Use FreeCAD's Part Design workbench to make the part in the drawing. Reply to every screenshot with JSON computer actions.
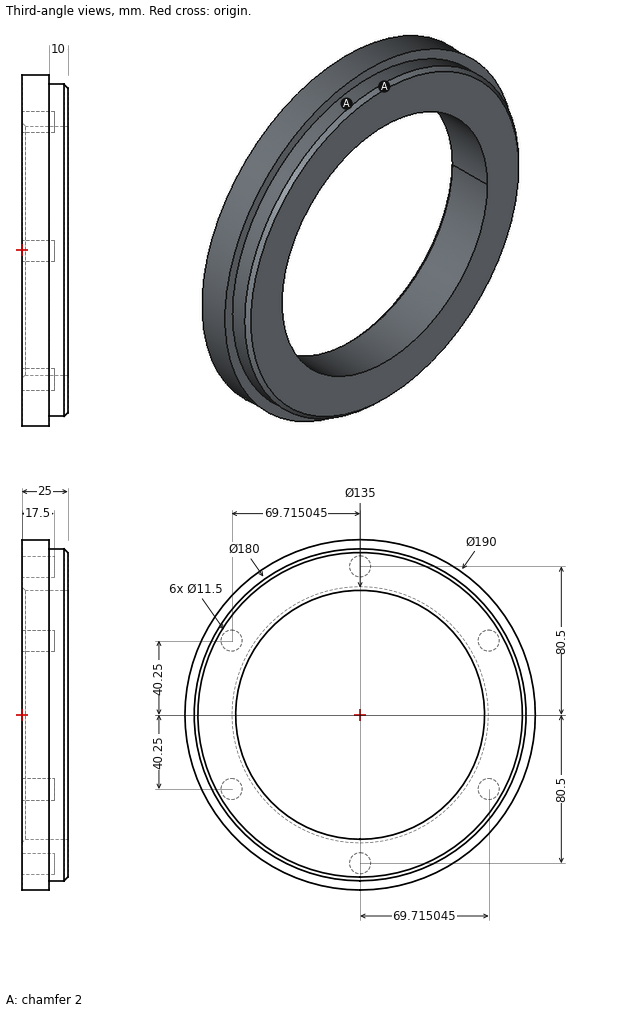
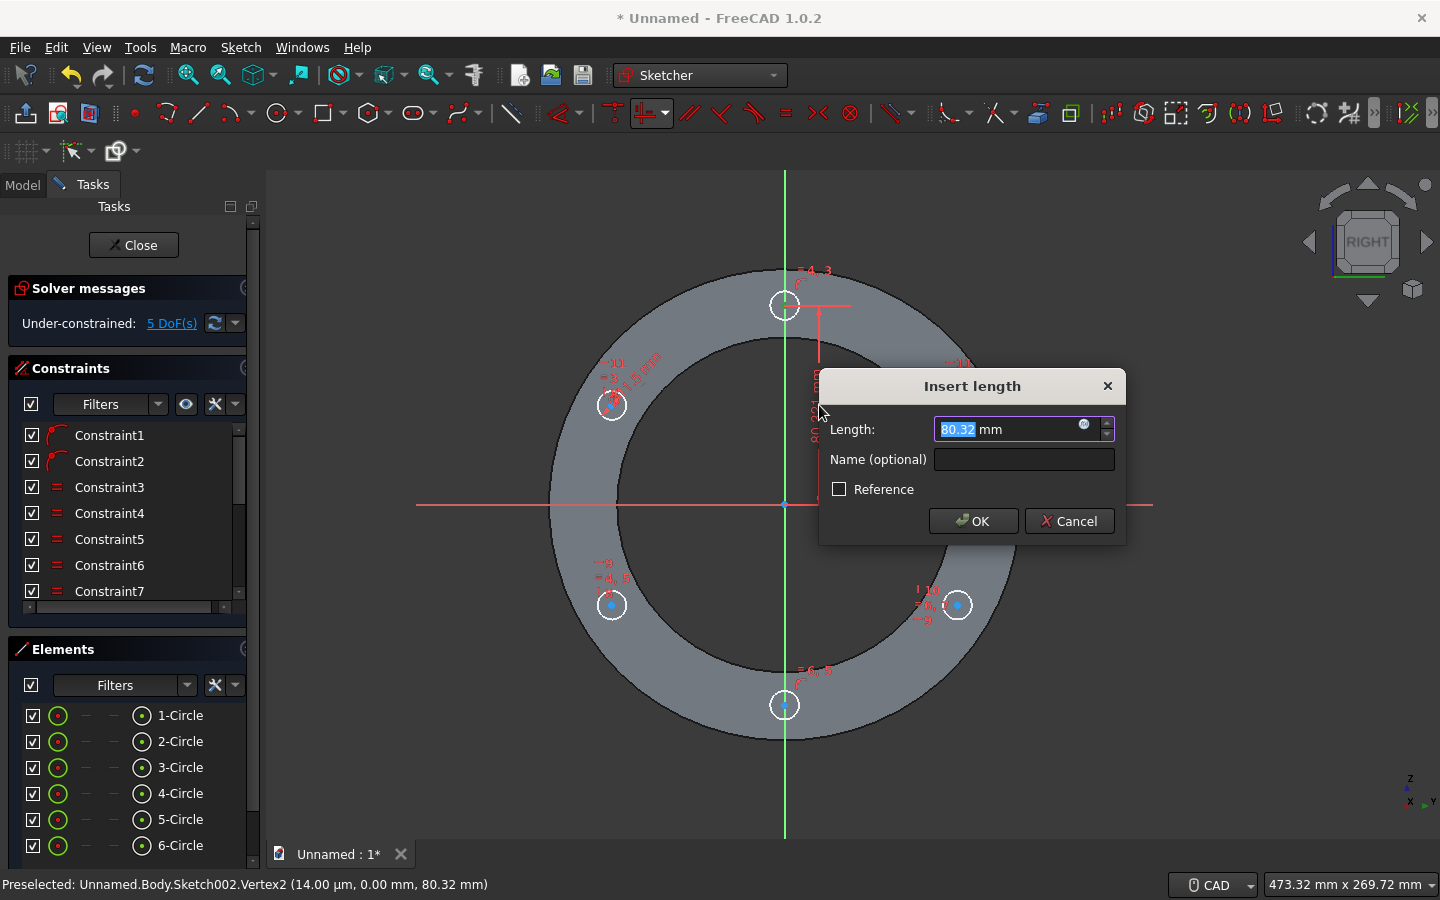
{"action": "type", "text": "80.5"}
{"action": "key", "text": "Return"}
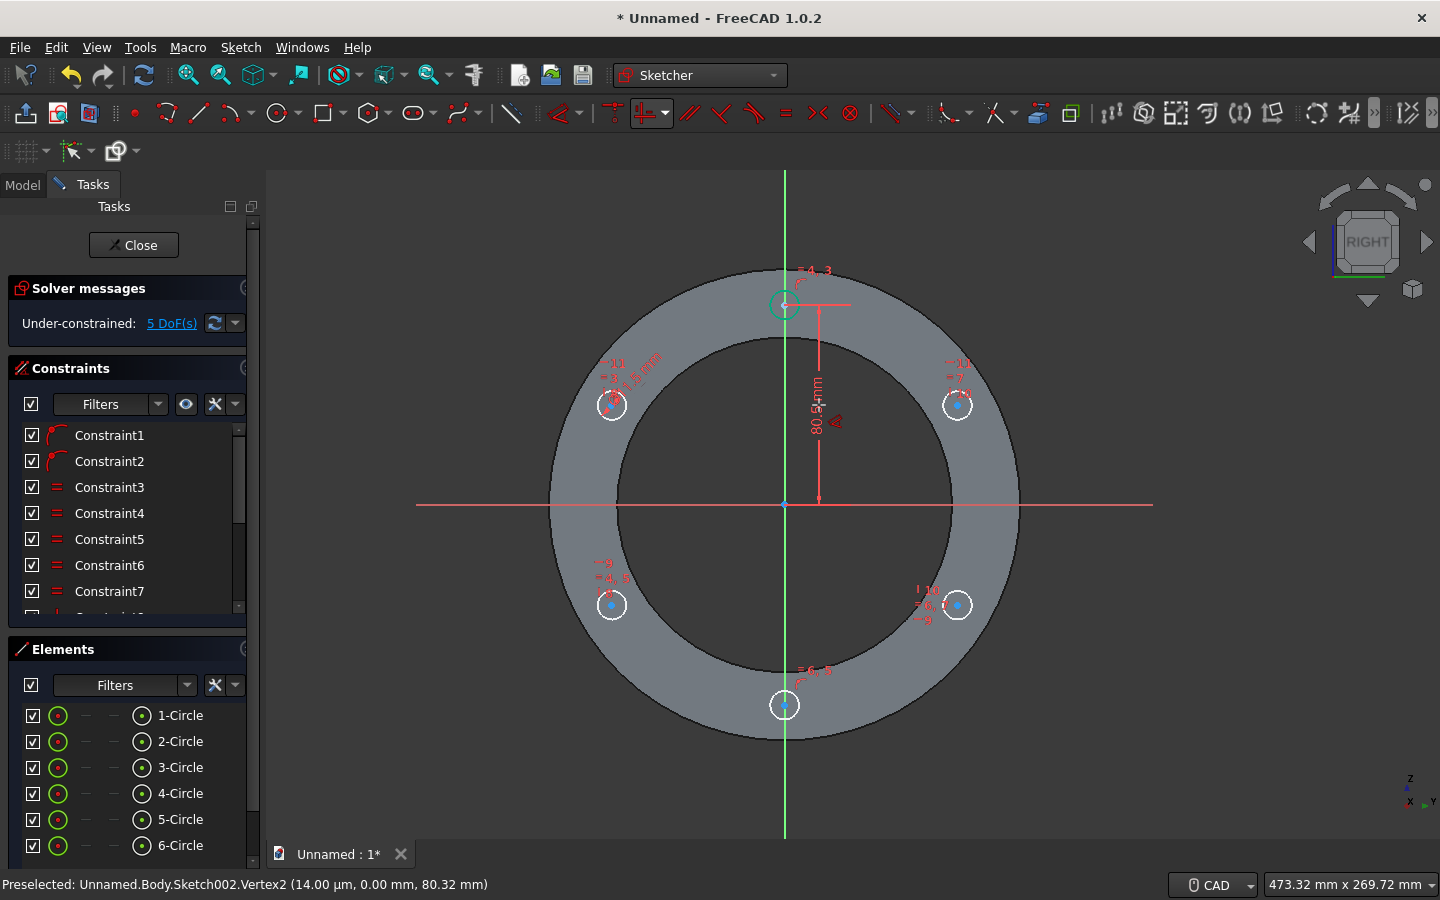
{"action": "left_click", "coordinate": [785, 705]}
{"action": "left_click", "coordinate": [819, 605]}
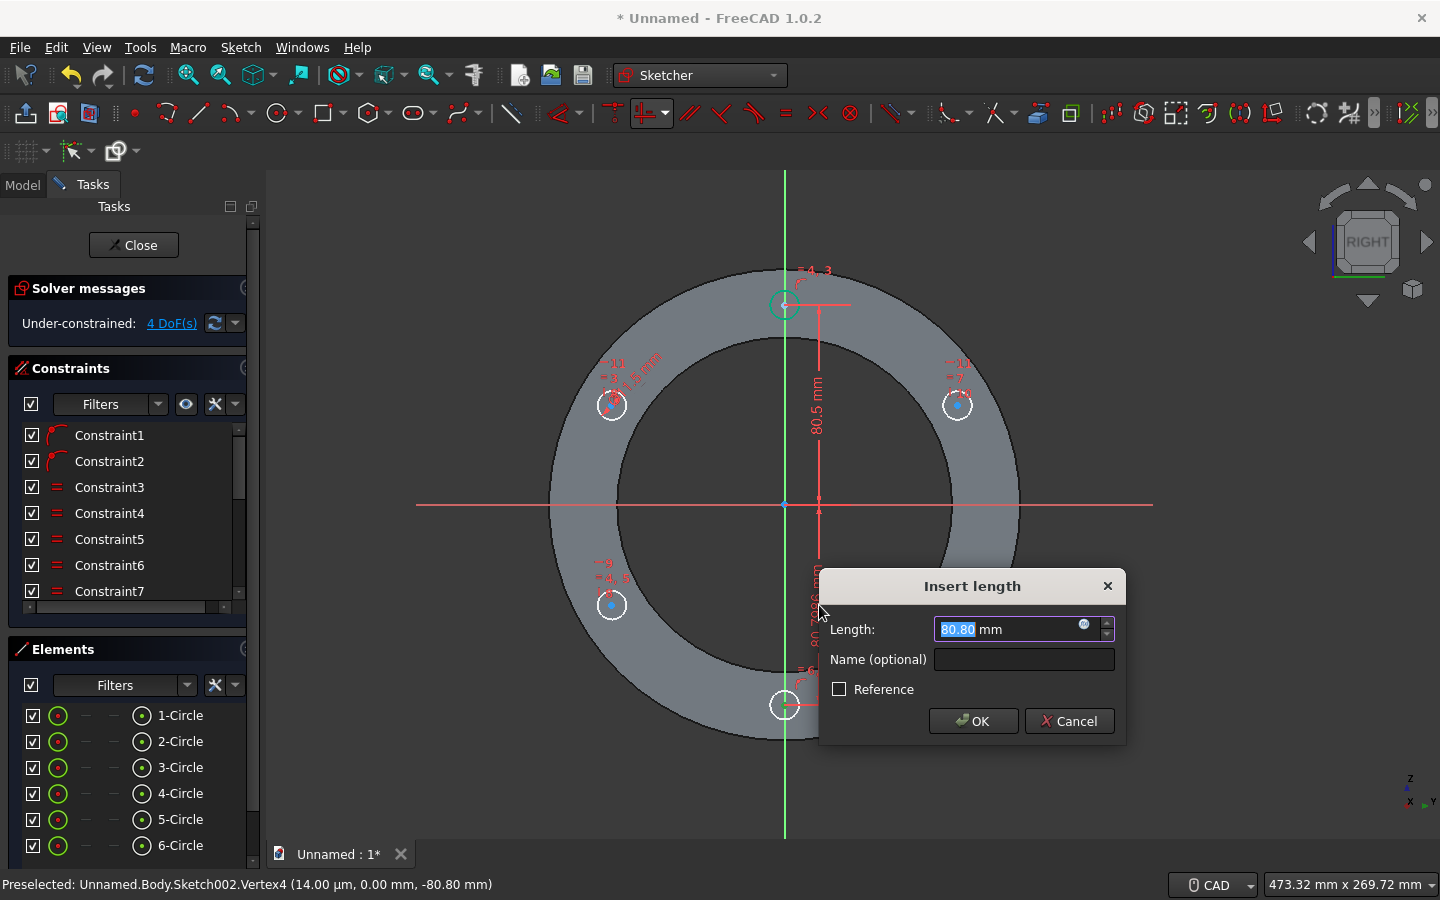
{"action": "type", "text": "80.5"}
{"action": "key", "text": "Return"}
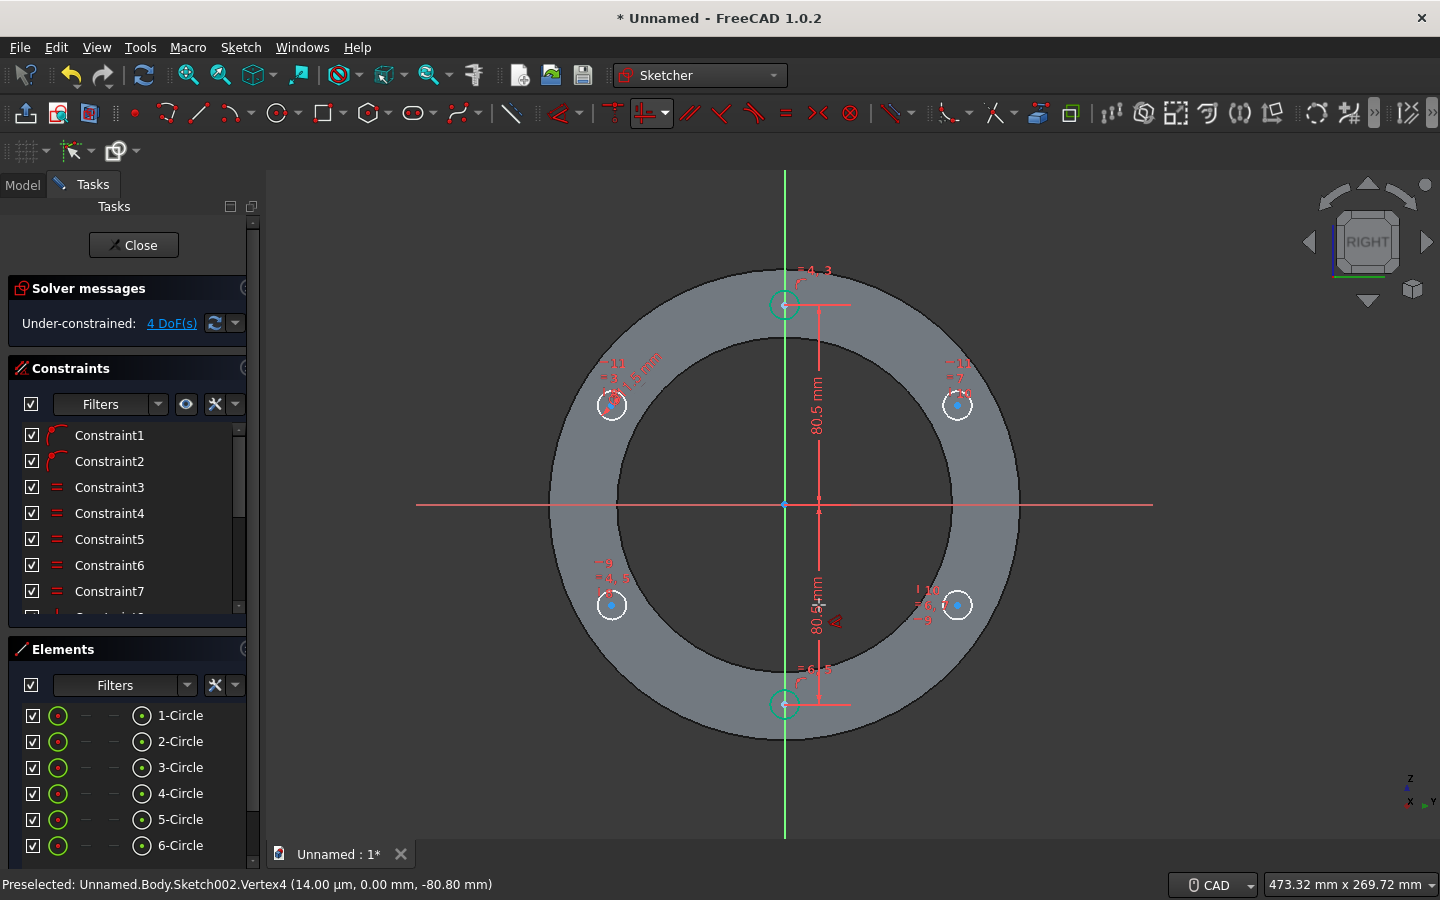
{"action": "left_click", "coordinate": [612, 405]}
{"action": "left_click", "coordinate": [578, 455]}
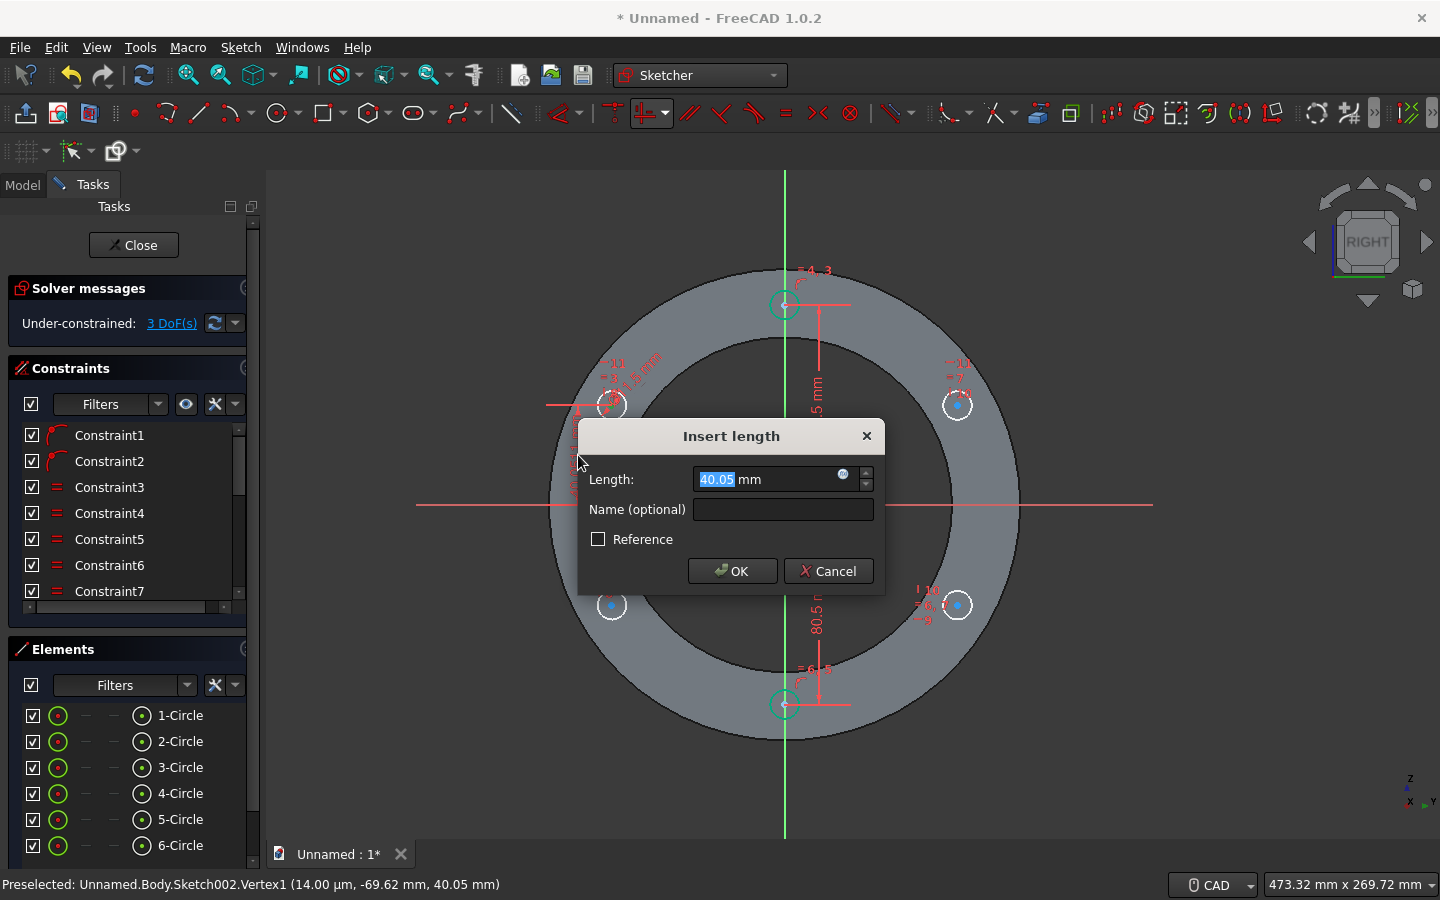
{"action": "type", "text": "40.25"}
{"action": "key", "text": "Return"}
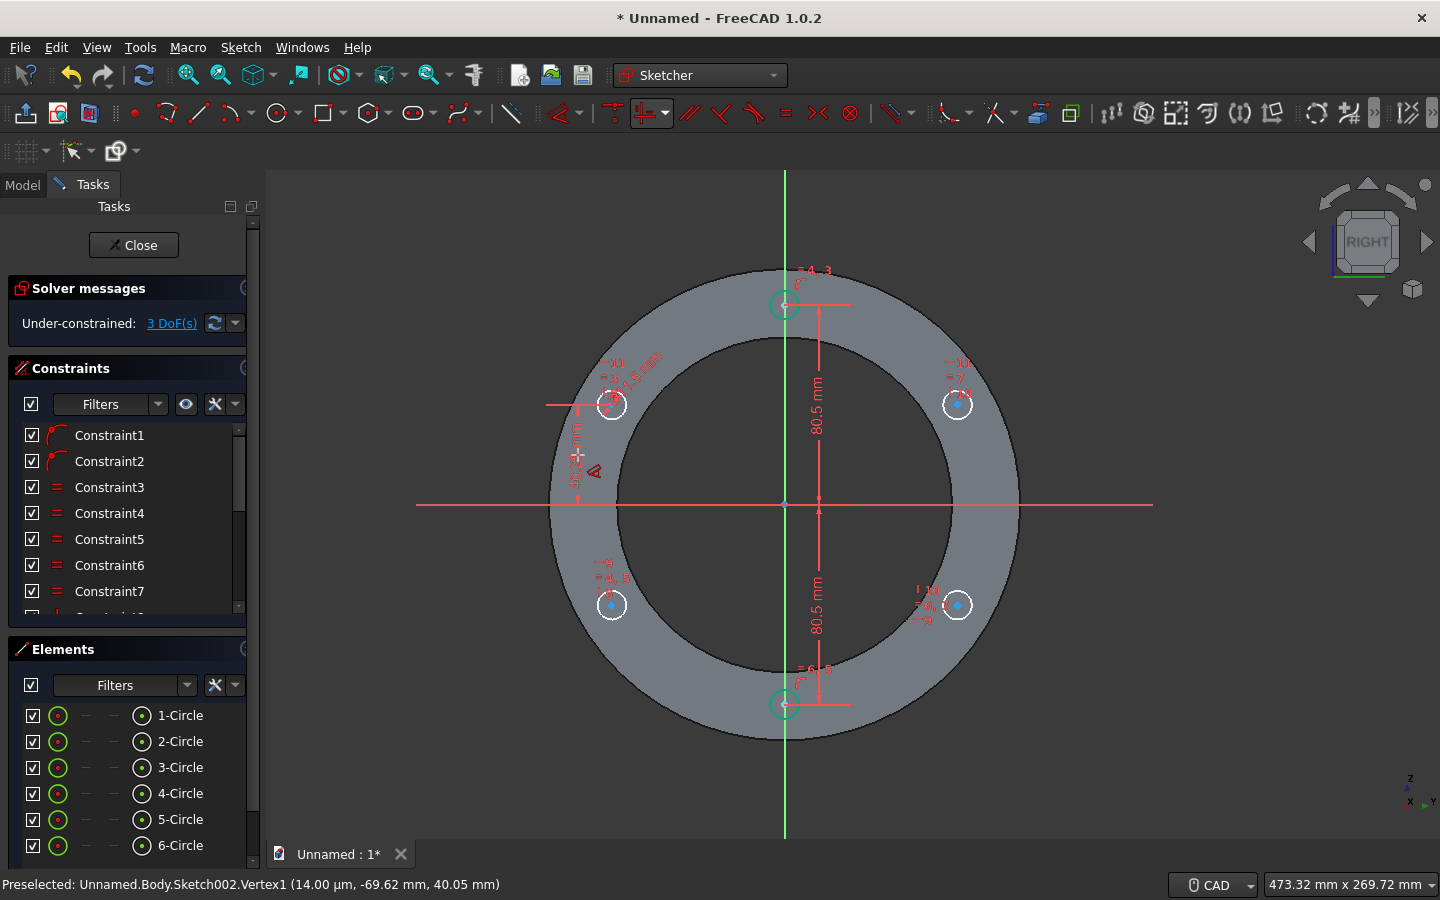
{"action": "left_click", "coordinate": [612, 605]}
{"action": "left_click", "coordinate": [578, 555]}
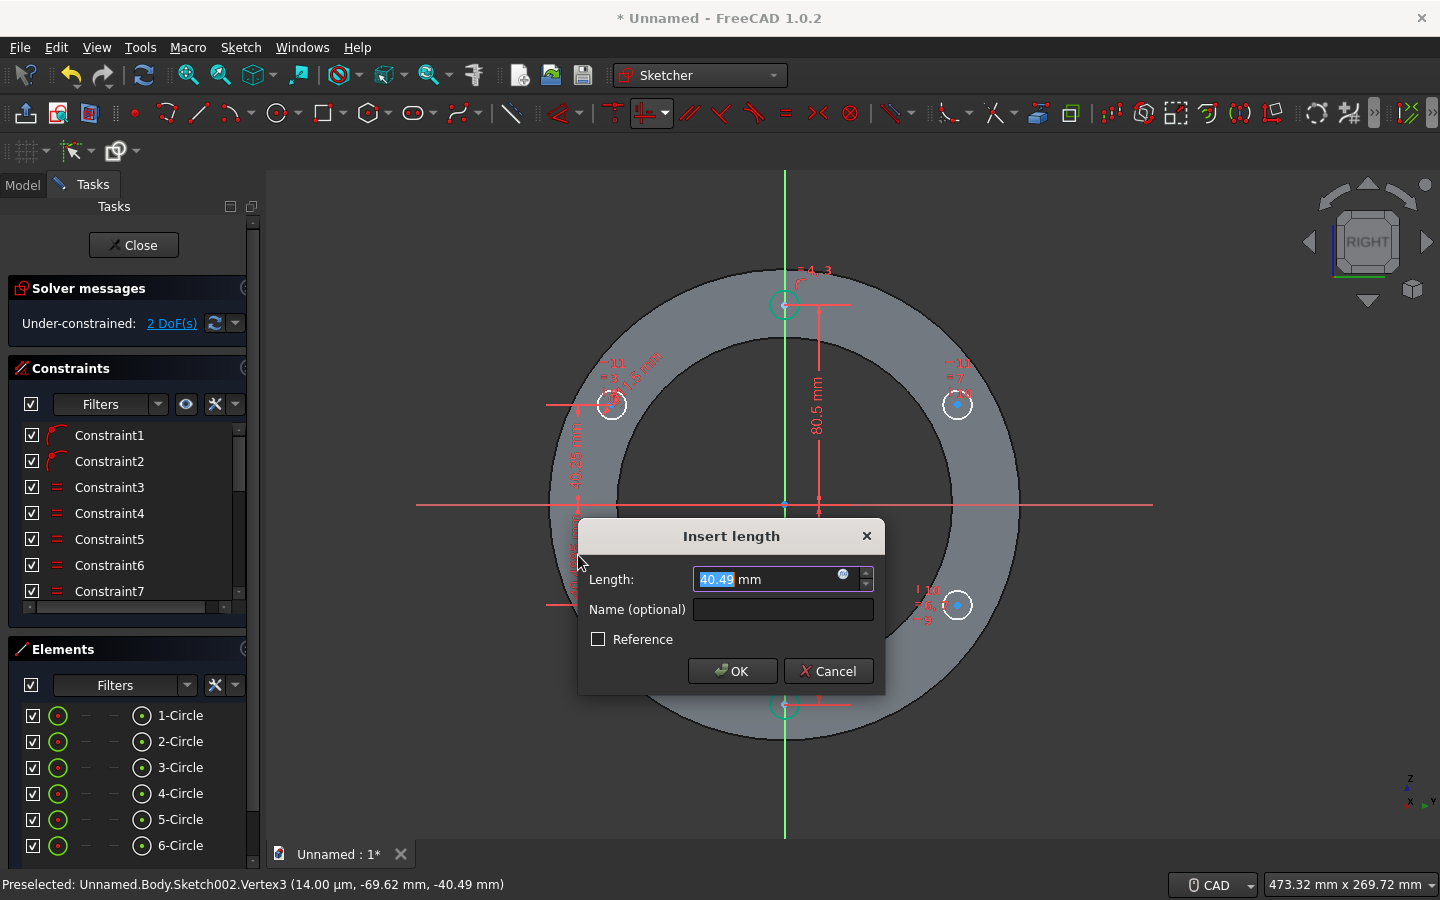
{"action": "type", "text": "40.25"}
{"action": "key", "text": "Return"}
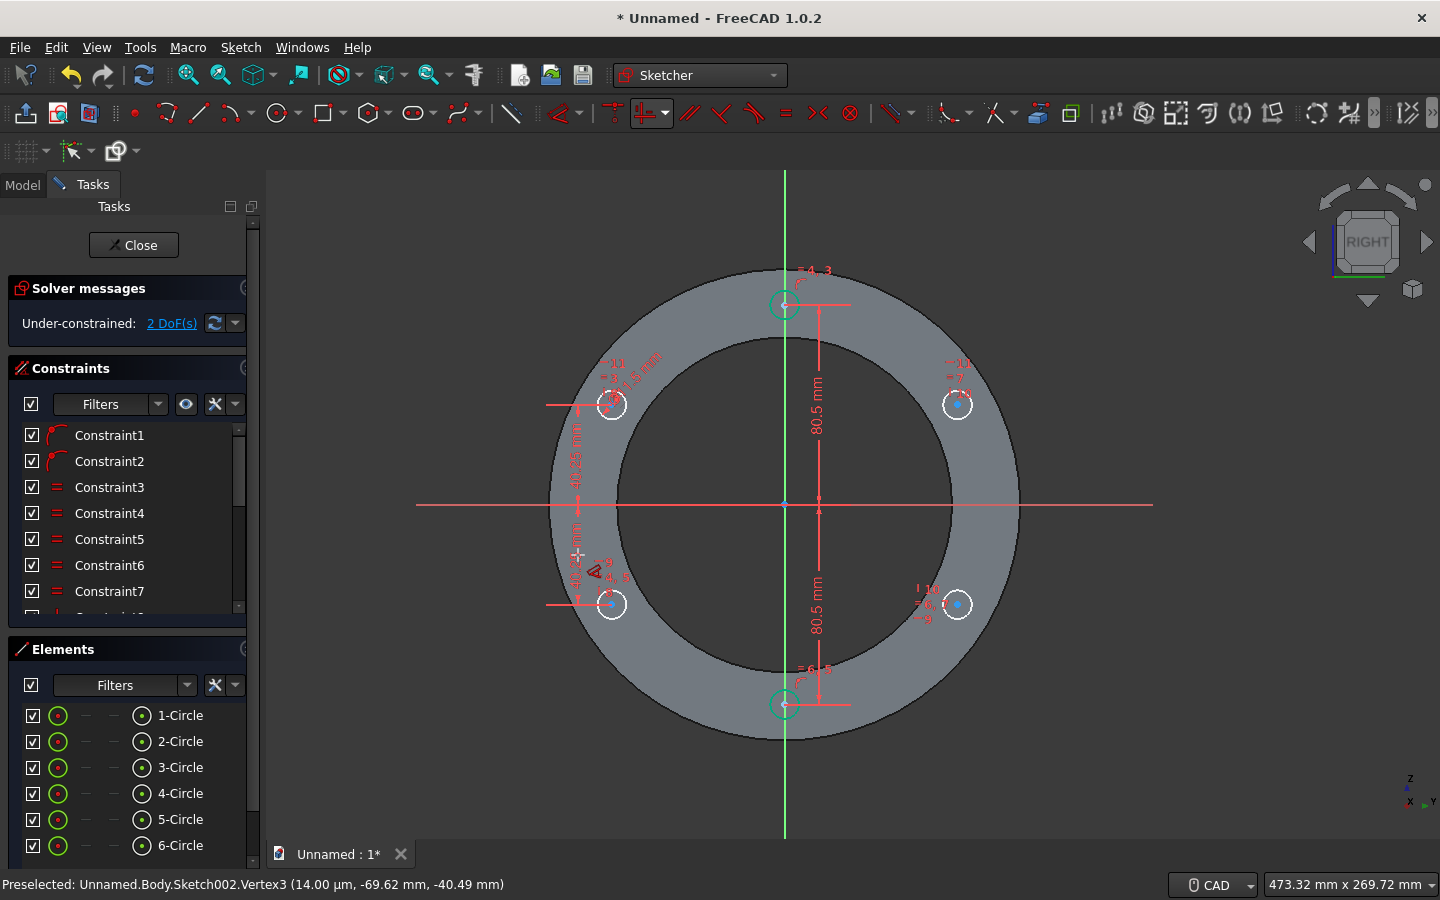
{"action": "left_click", "coordinate": [612, 405]}
{"action": "left_click", "coordinate": [738, 371]}